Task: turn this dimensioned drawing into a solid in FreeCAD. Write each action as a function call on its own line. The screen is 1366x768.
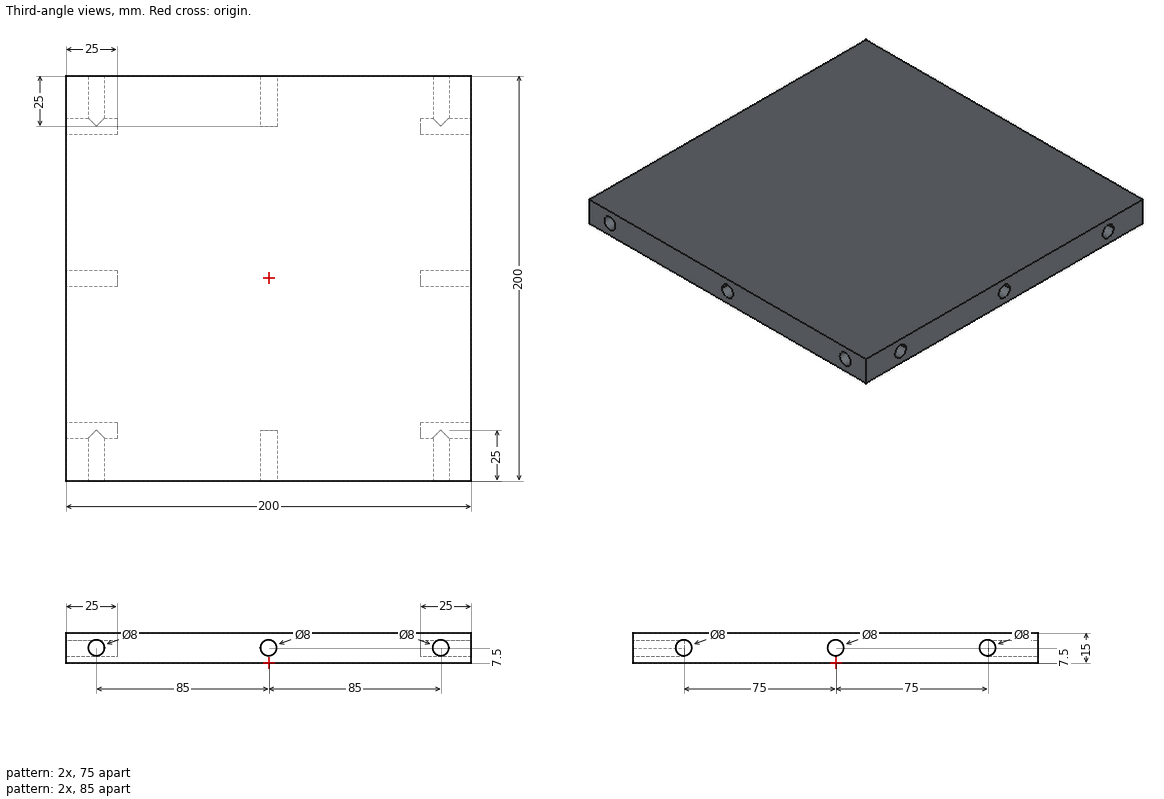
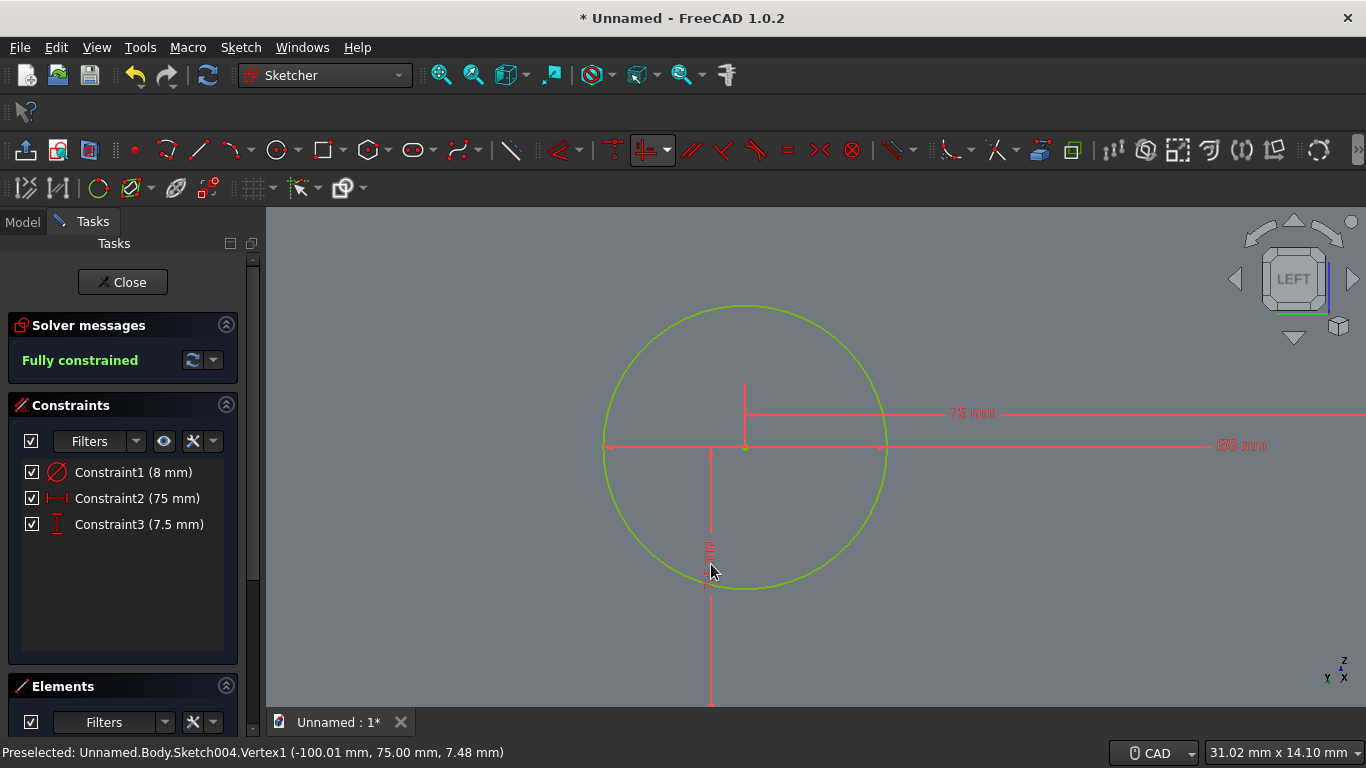
click(123, 282)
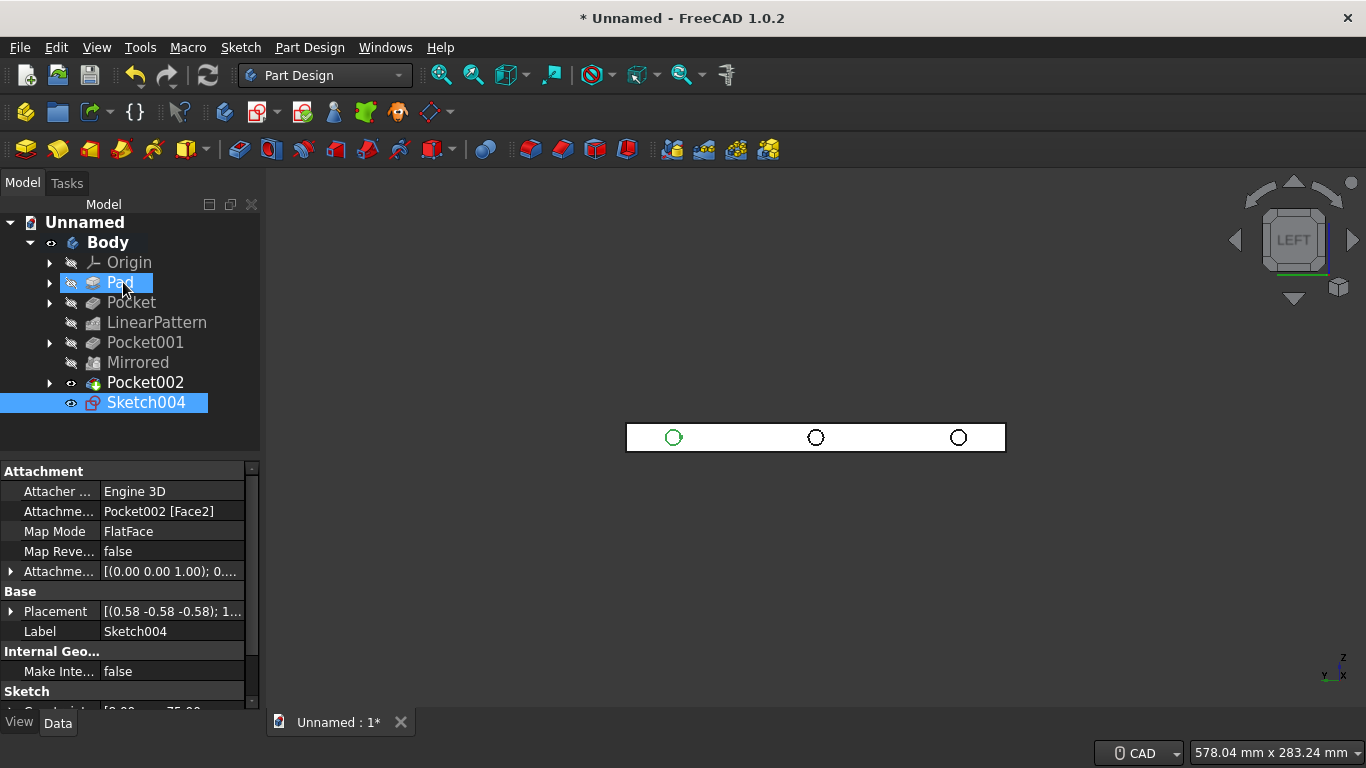
click(240, 150)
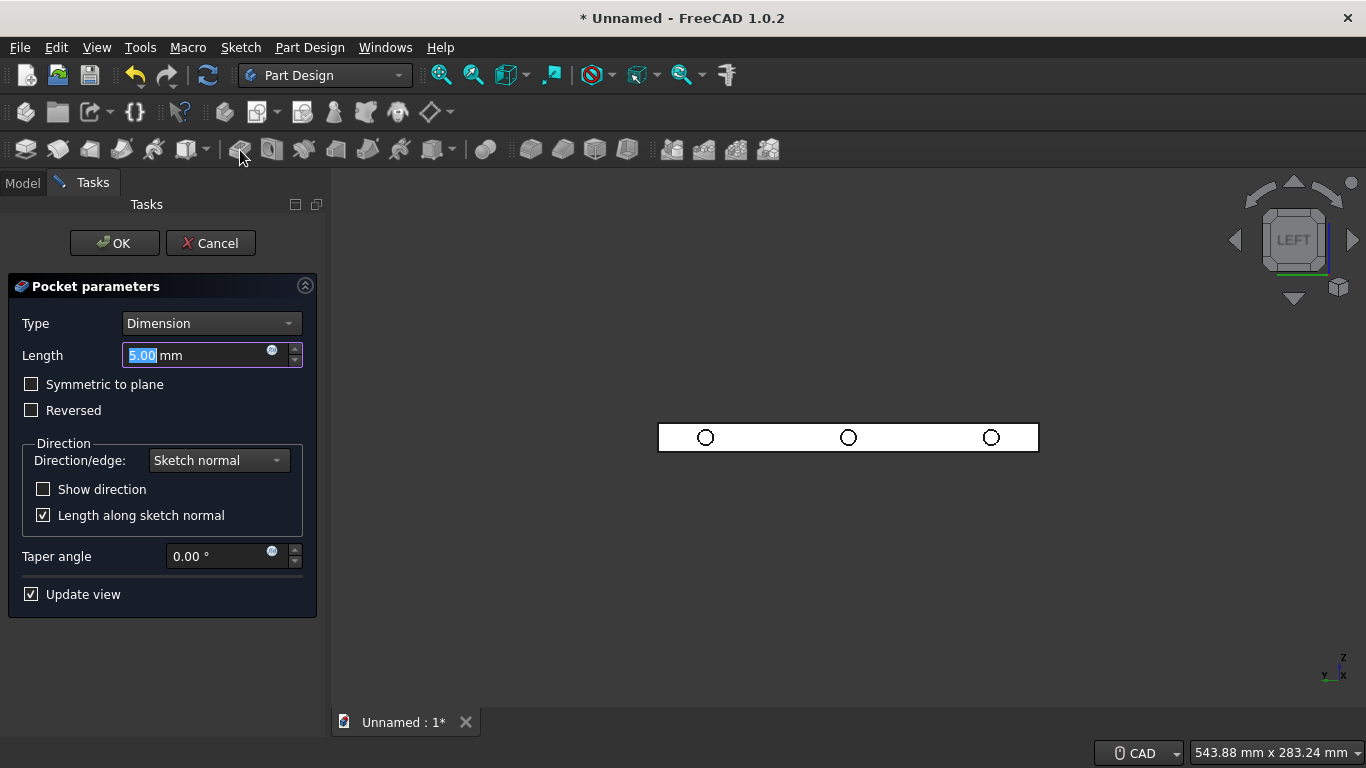
text(25)
key(Tab)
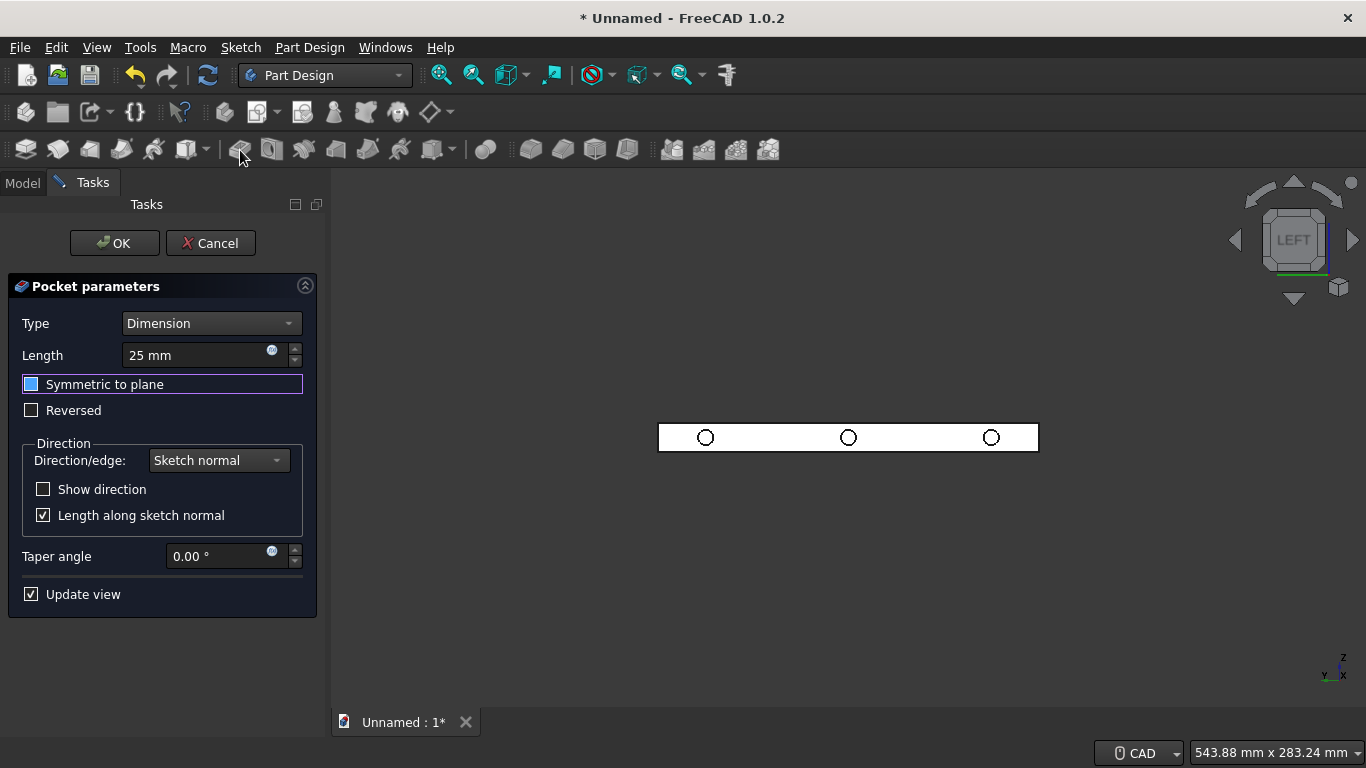
click(115, 243)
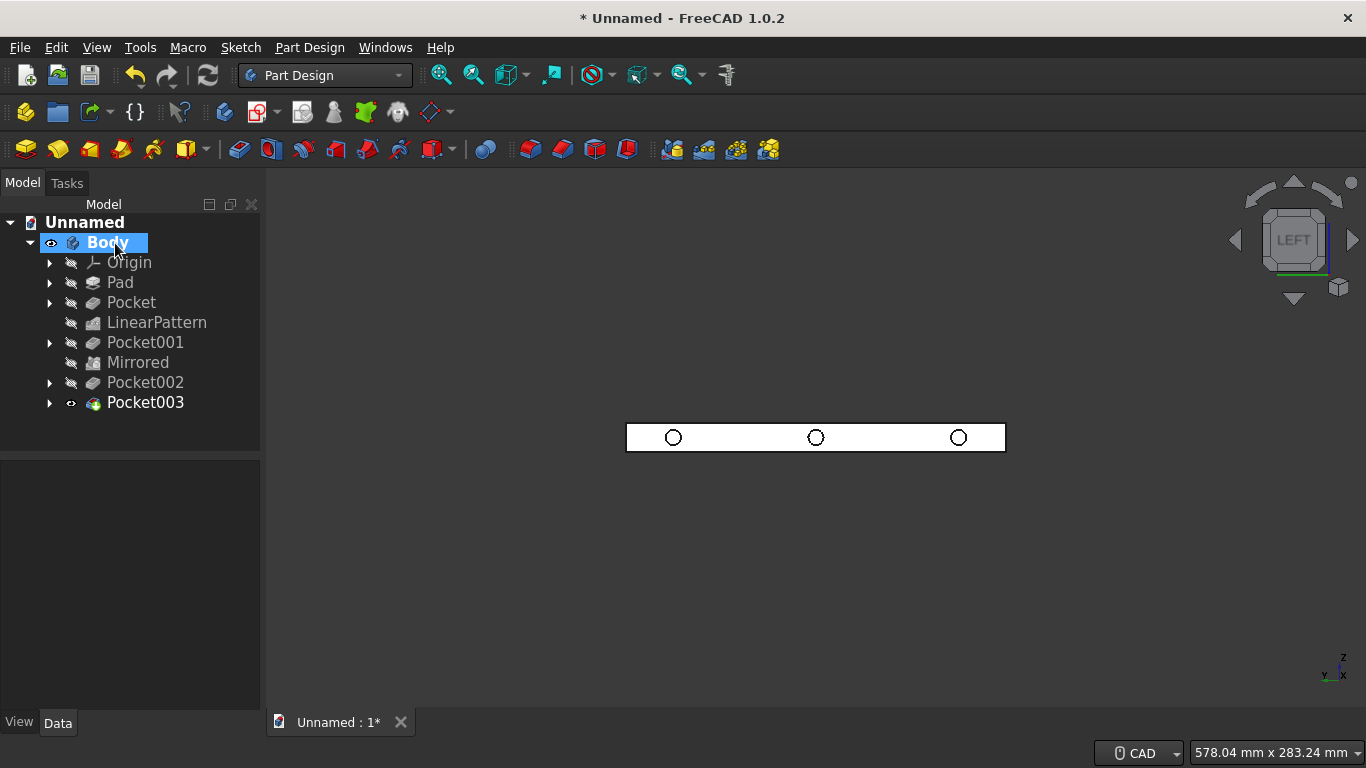
key(v)
key(f)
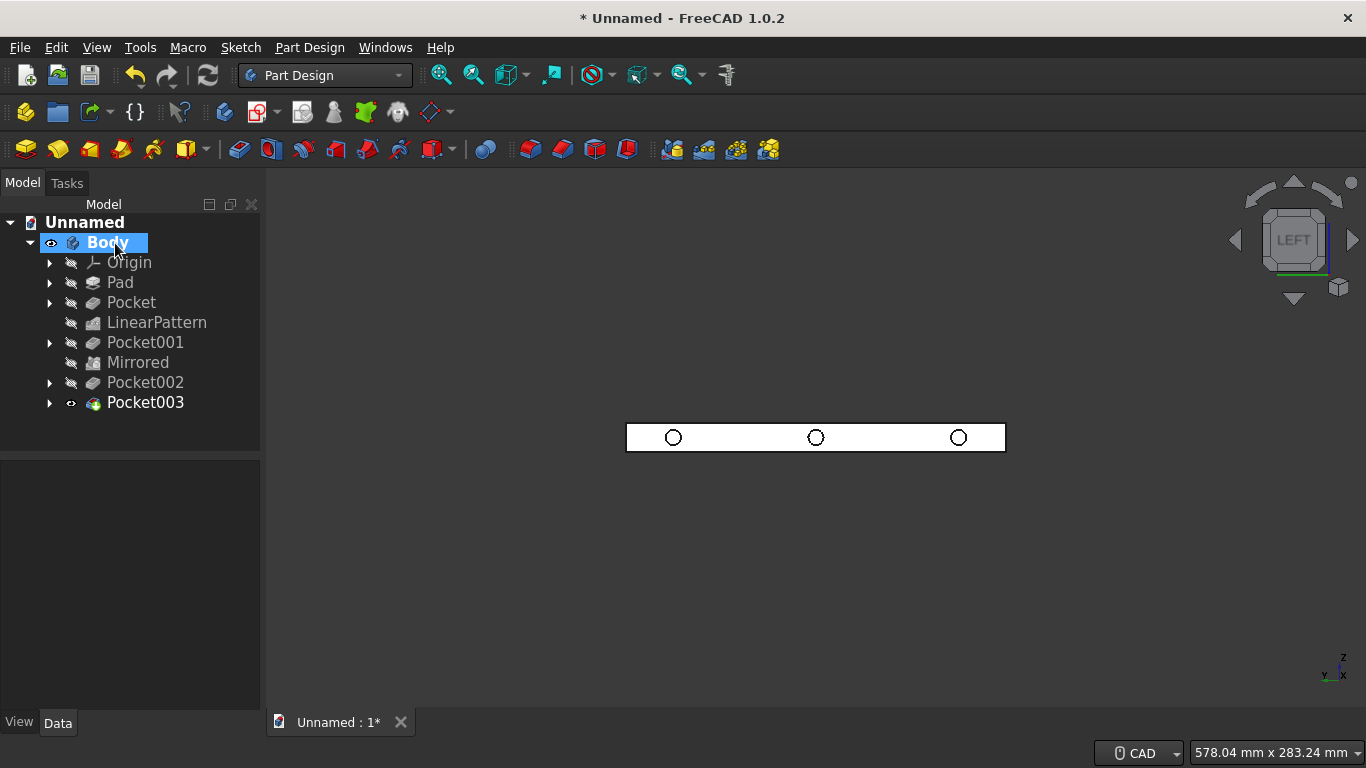
key(4)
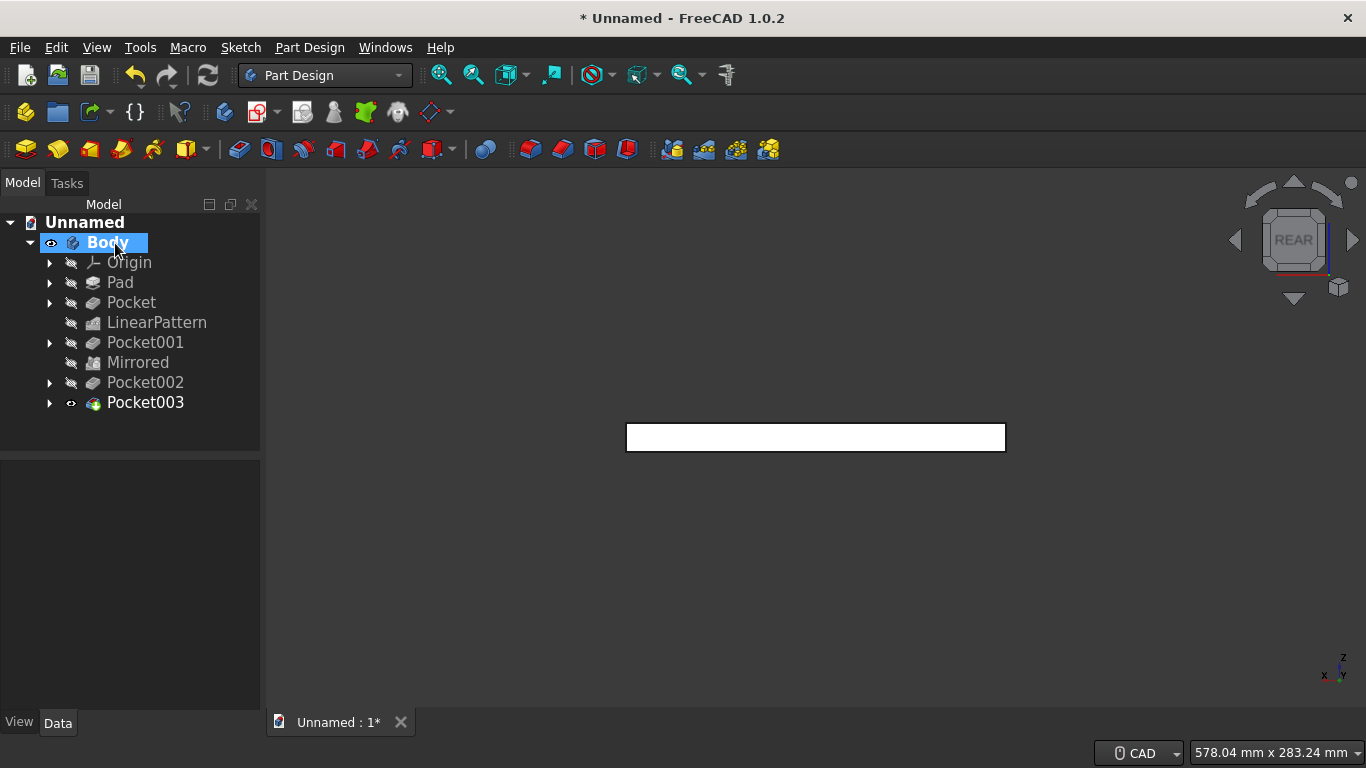
key(v)
key(f)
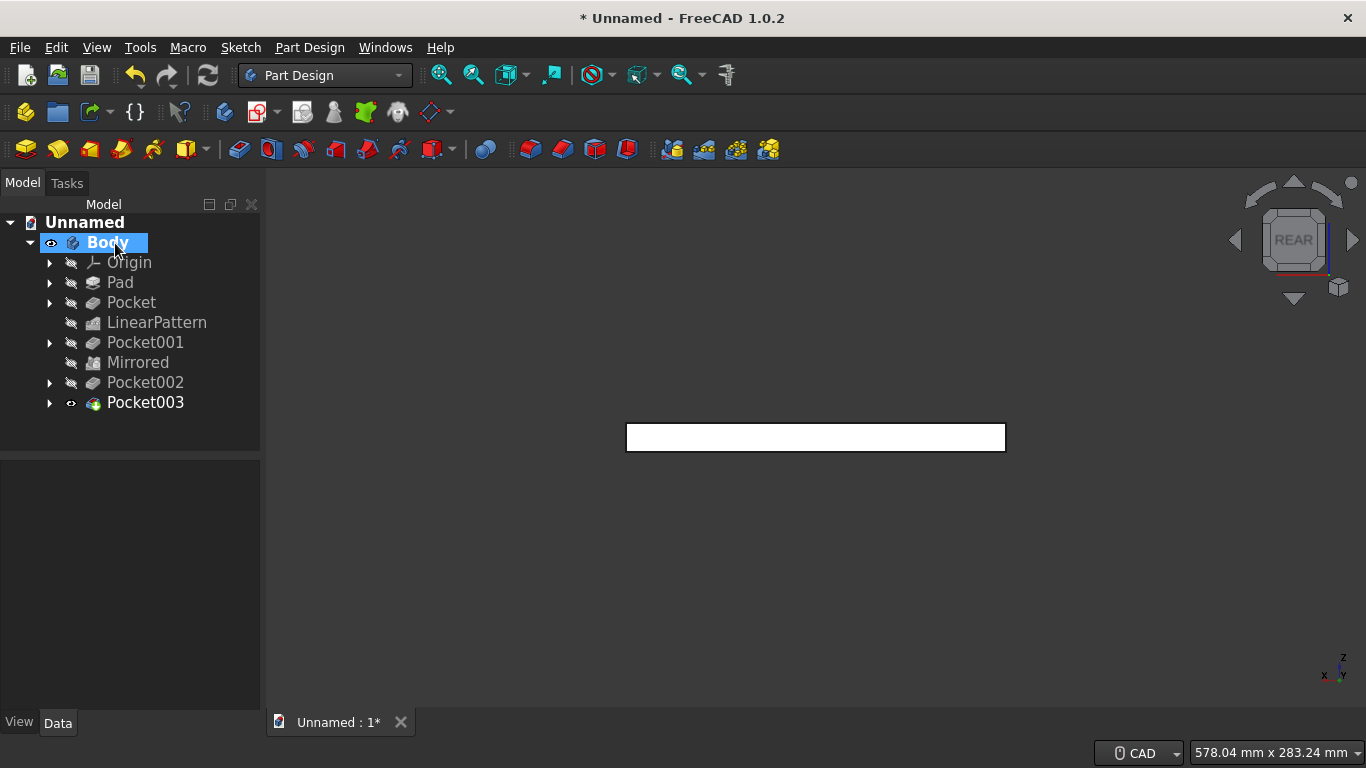
click(653, 437)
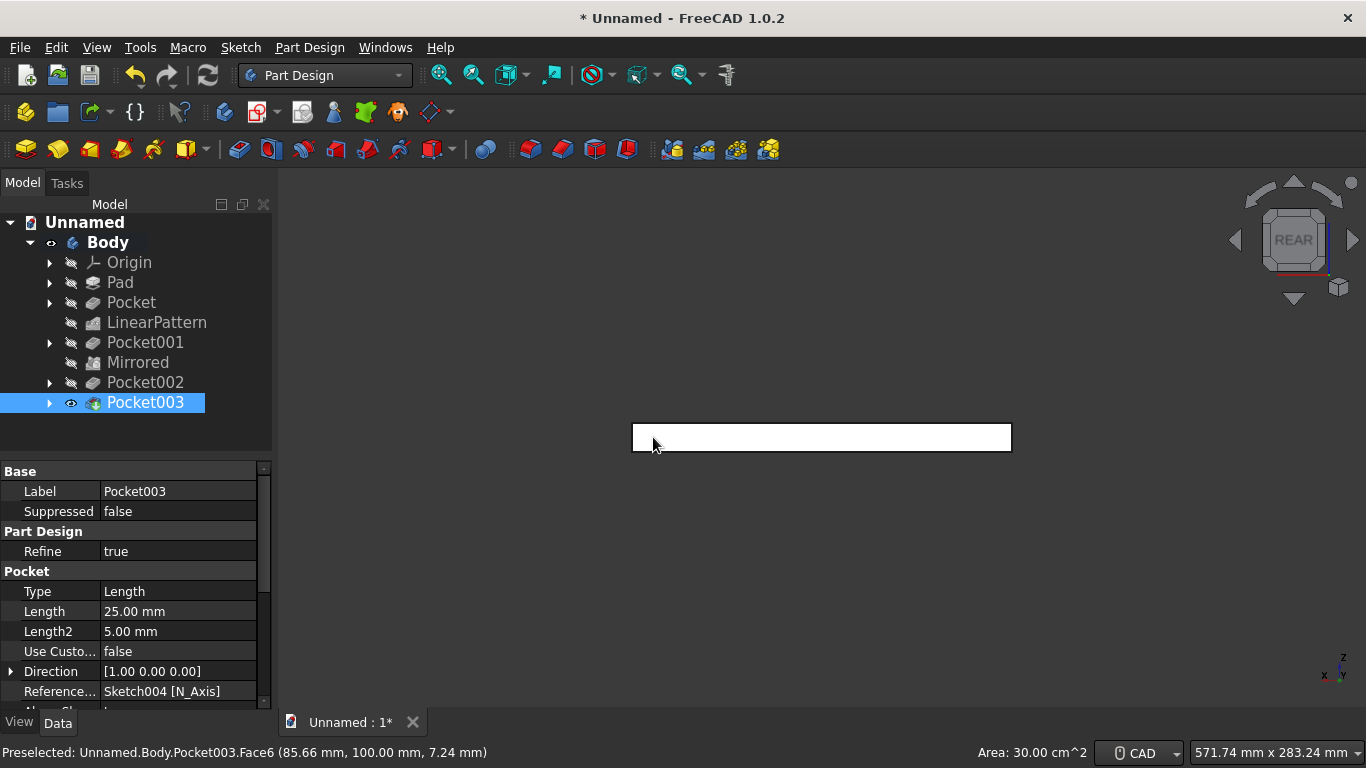
click(258, 112)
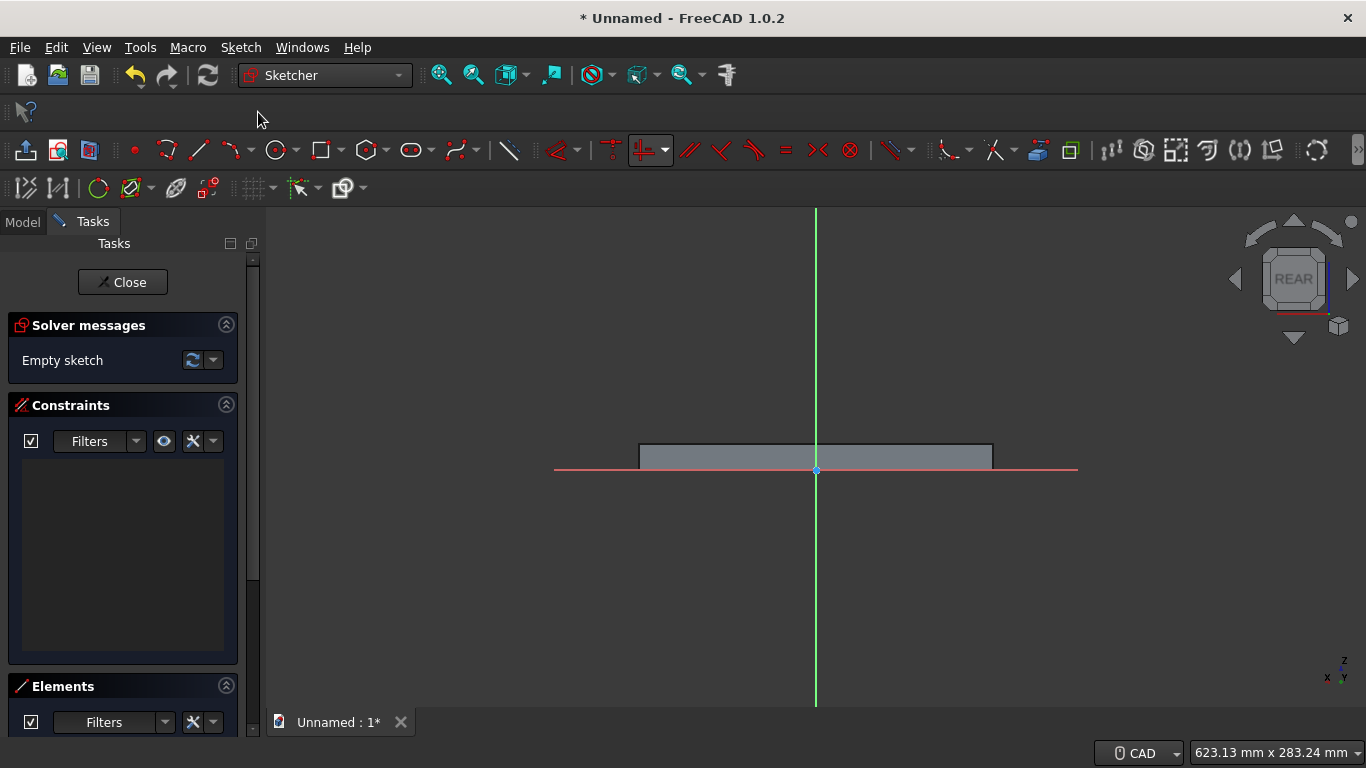
scroll(820, 460, up, 14)